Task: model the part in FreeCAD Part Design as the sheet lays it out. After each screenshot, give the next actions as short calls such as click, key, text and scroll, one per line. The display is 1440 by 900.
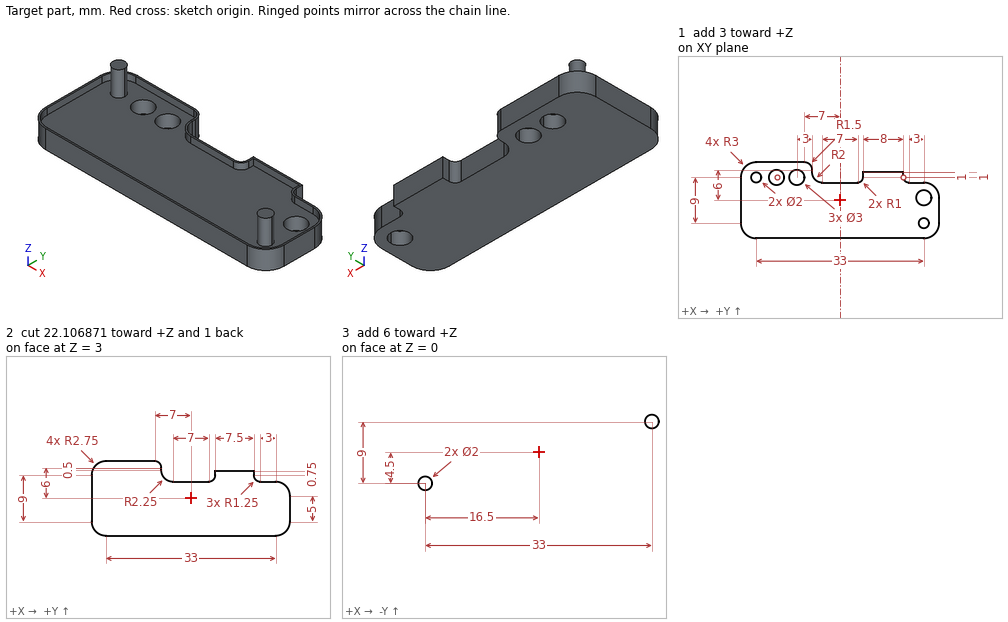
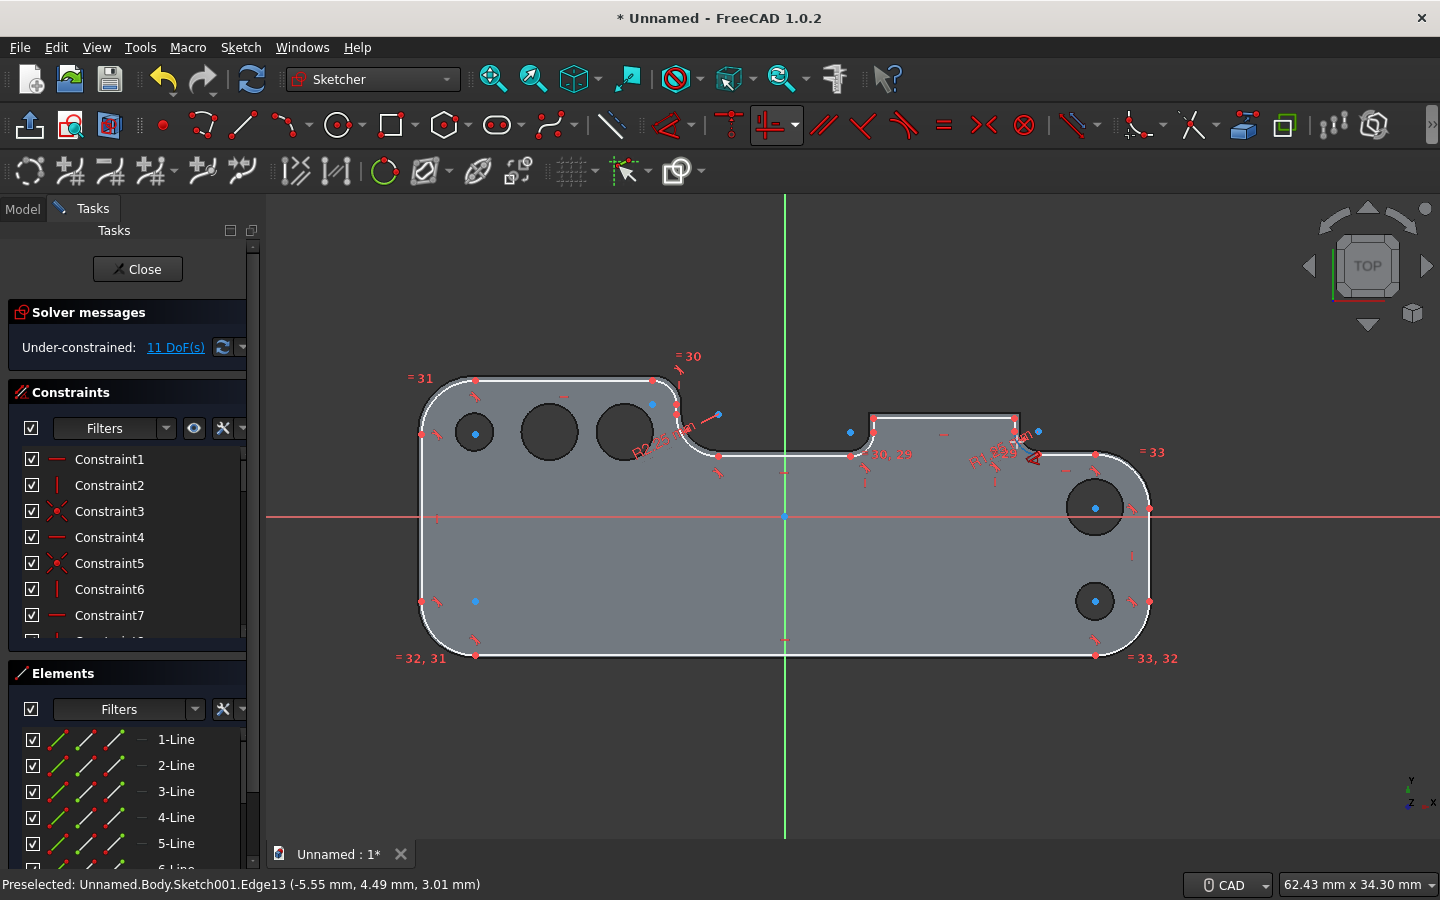
click(451, 387)
click(436, 359)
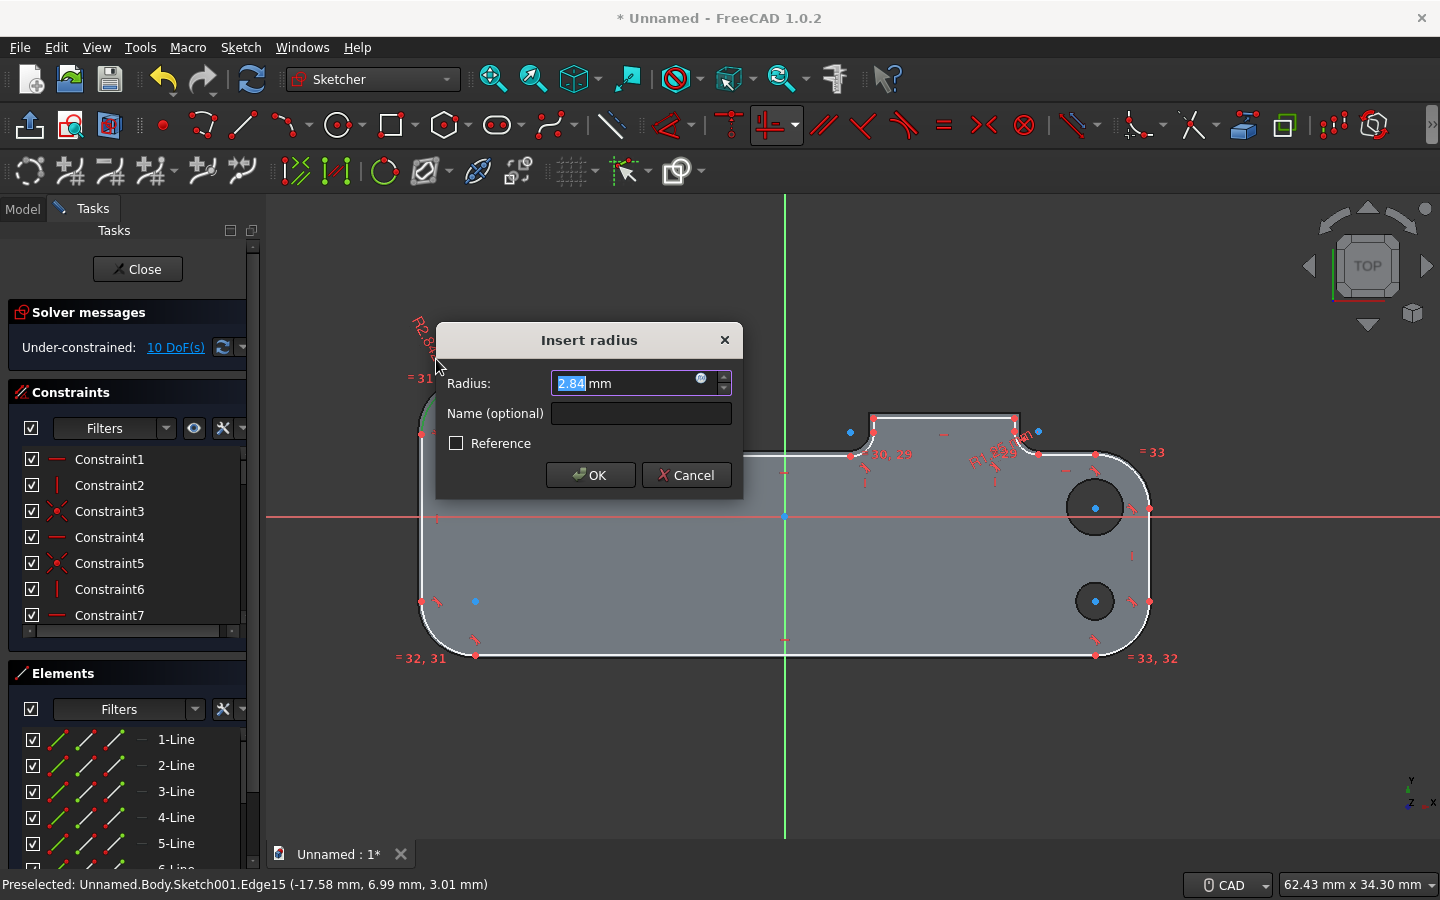
text(2.75)
key(Return)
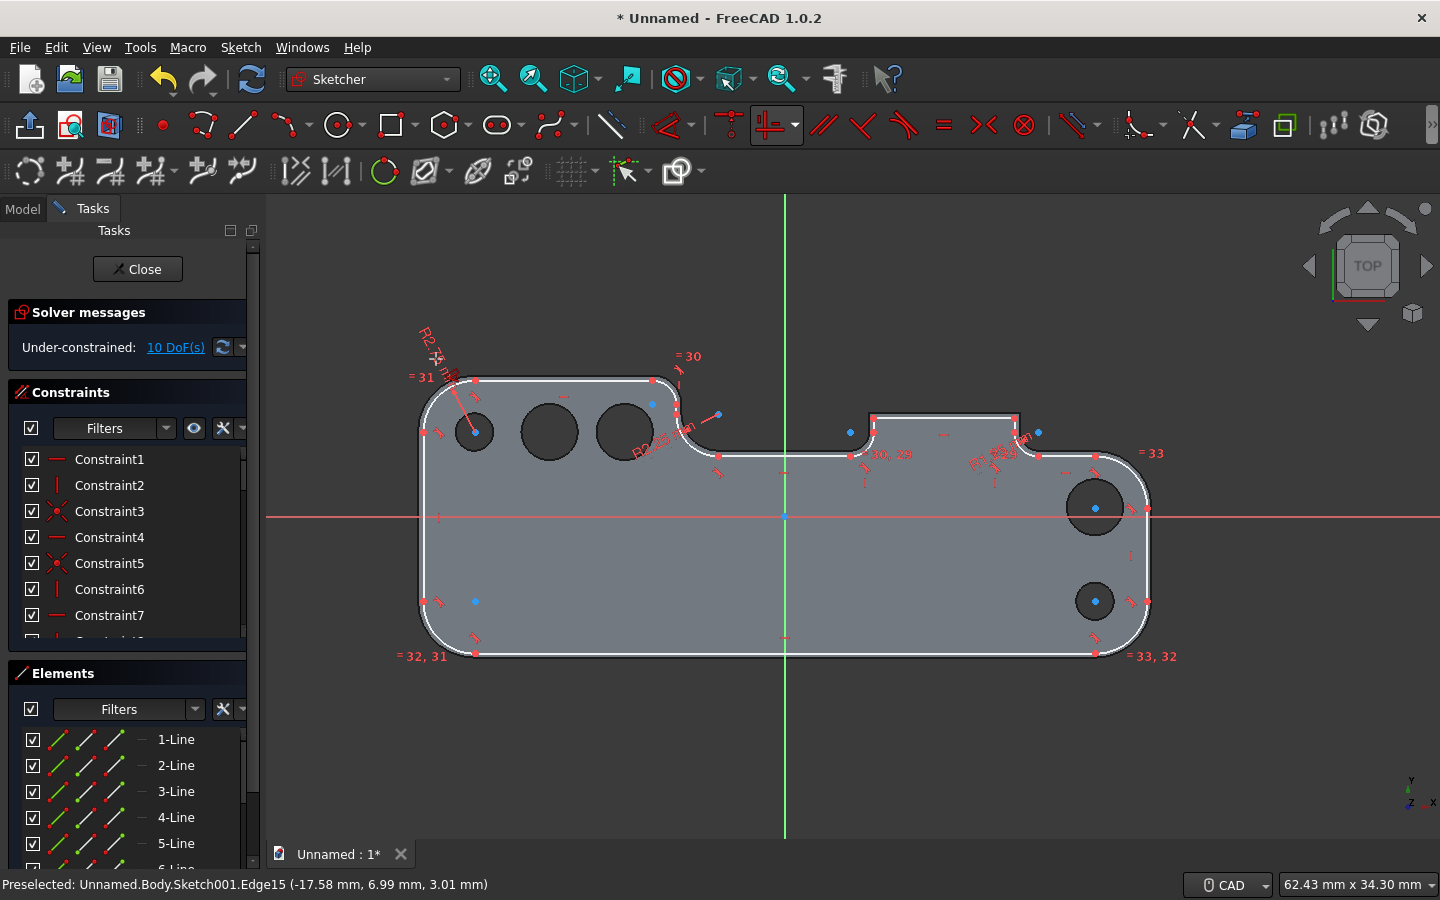
click(1078, 456)
click(1067, 422)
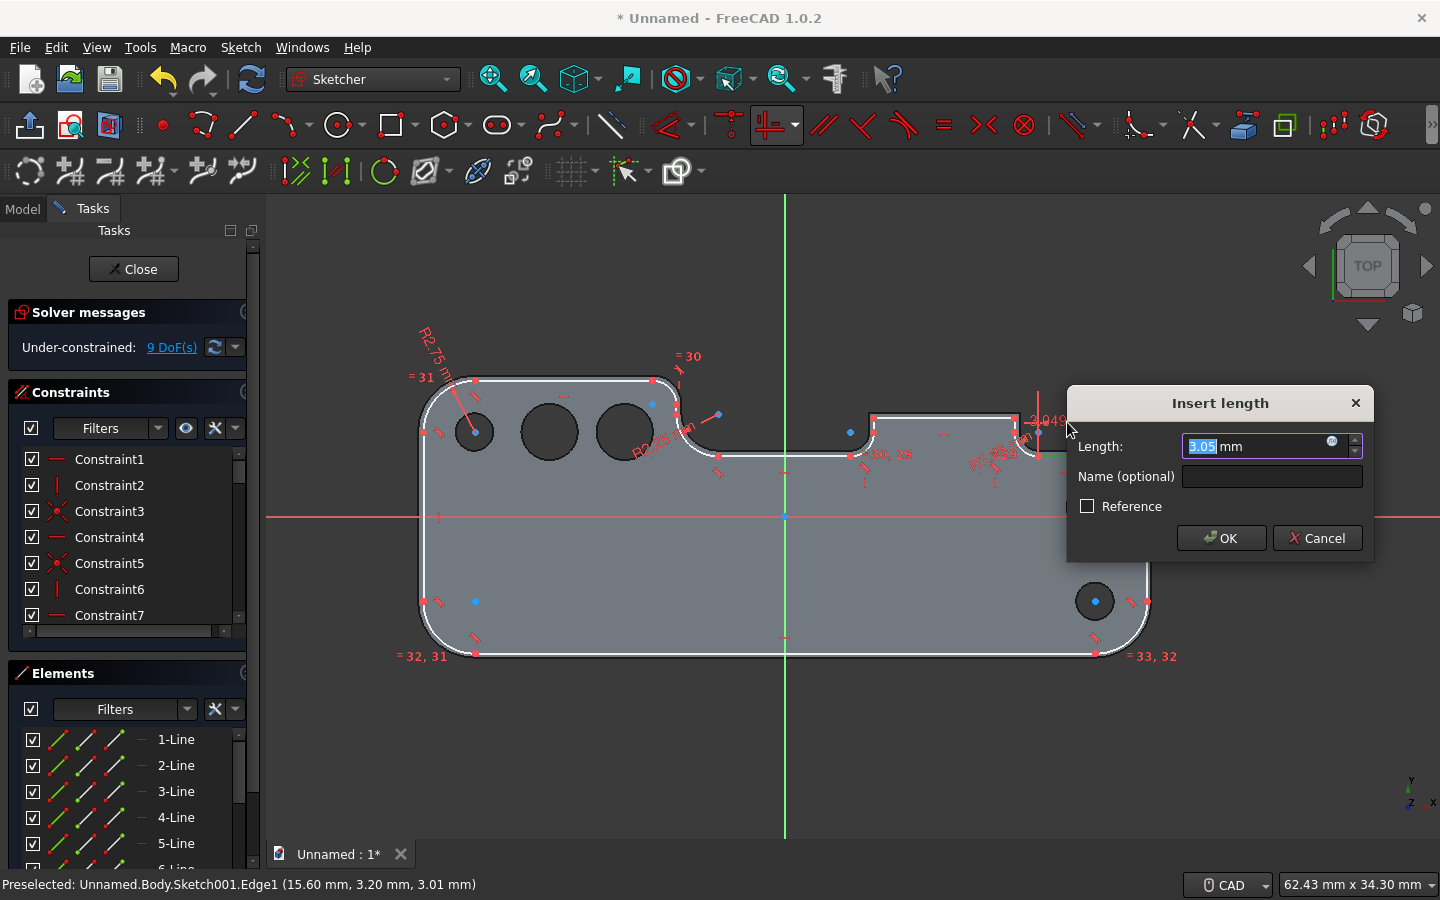
text(3)
key(Return)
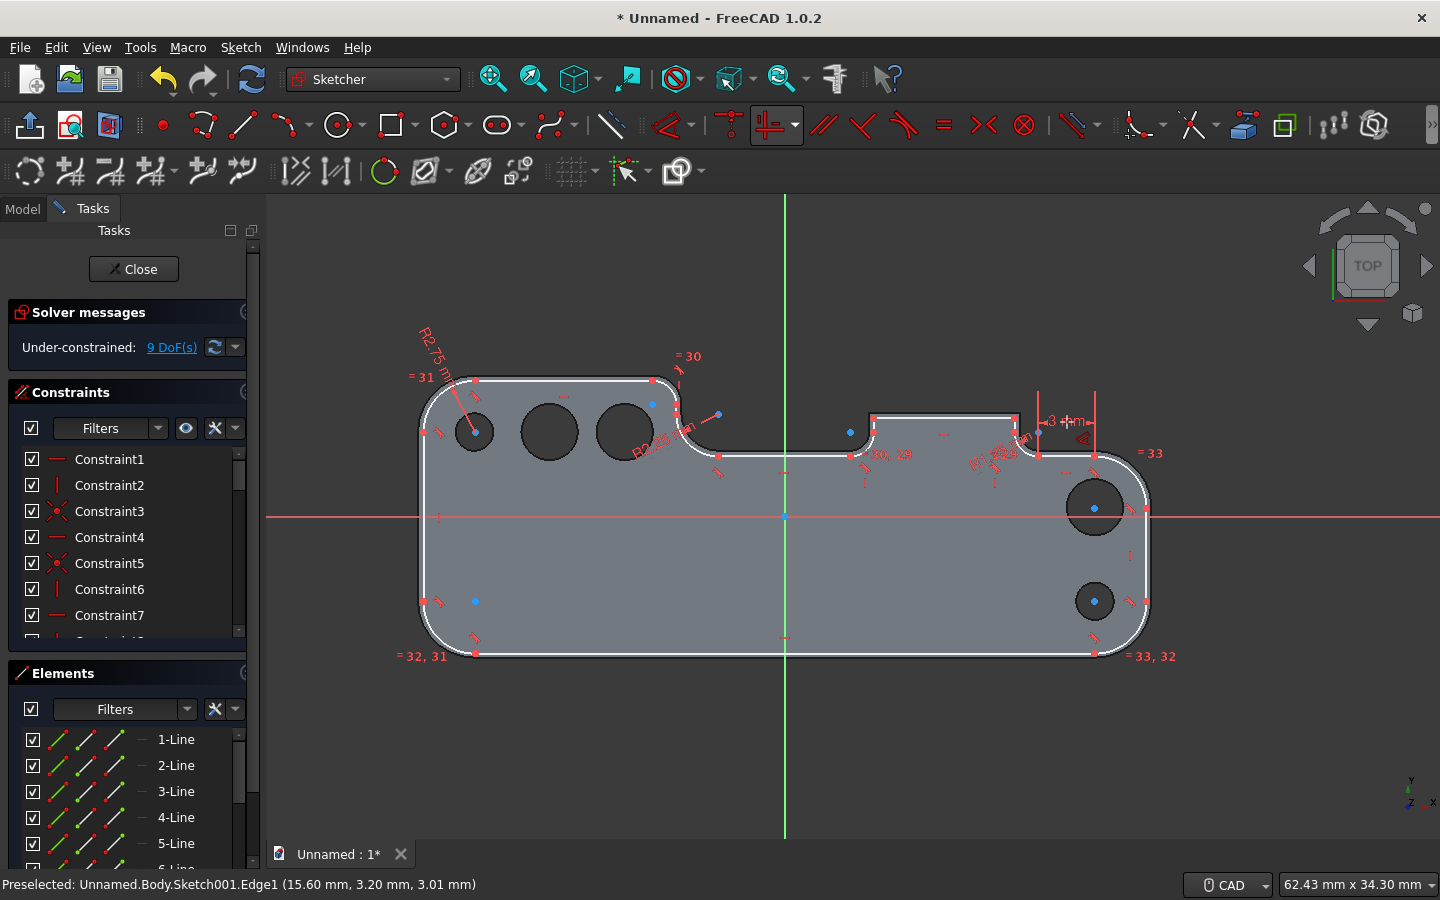
click(811, 456)
click(754, 422)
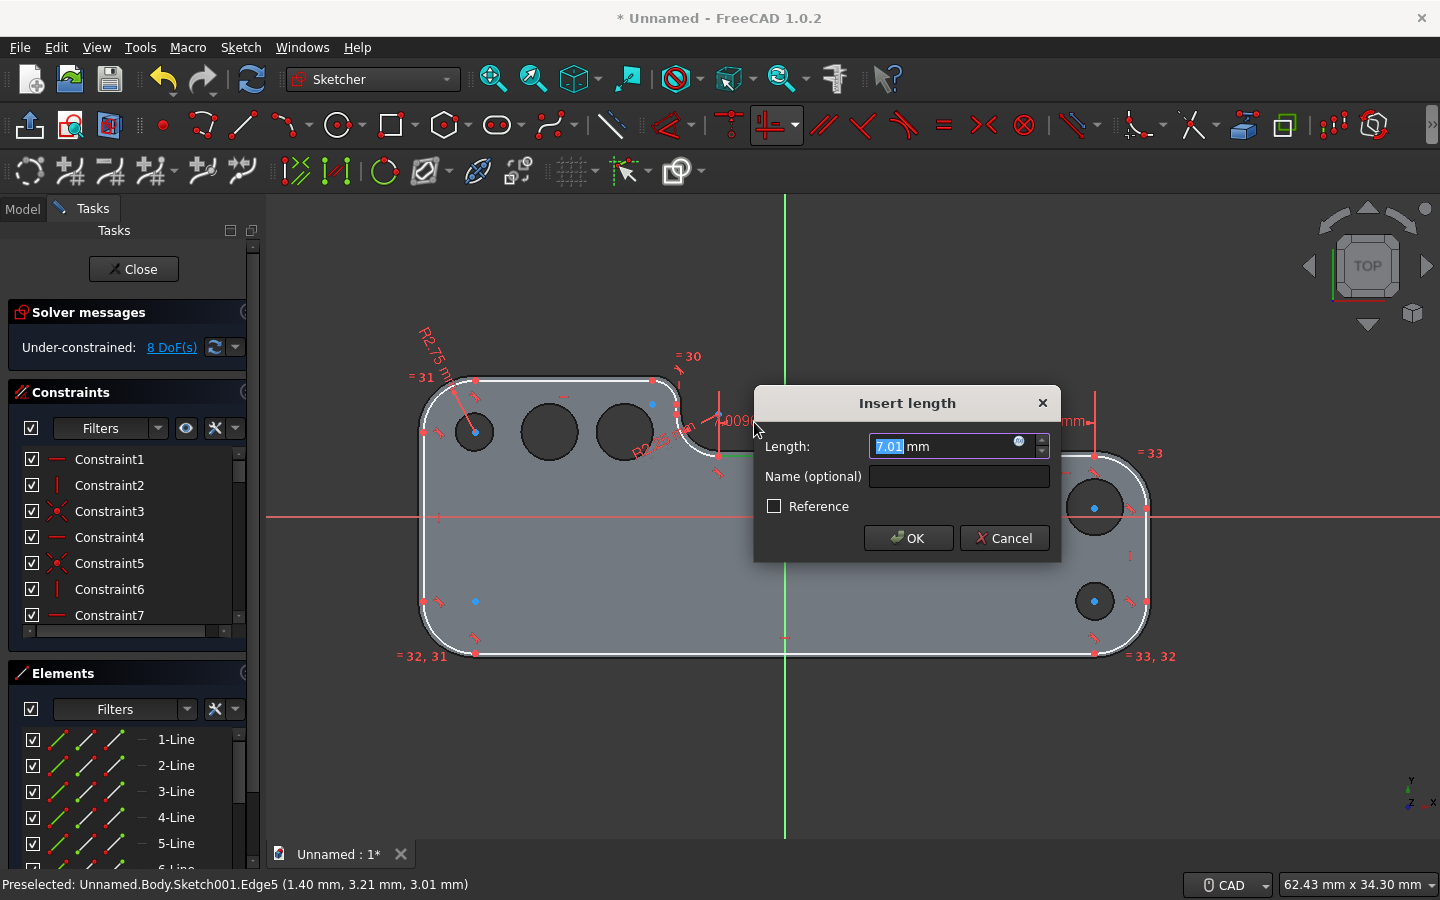
text(7)
key(Return)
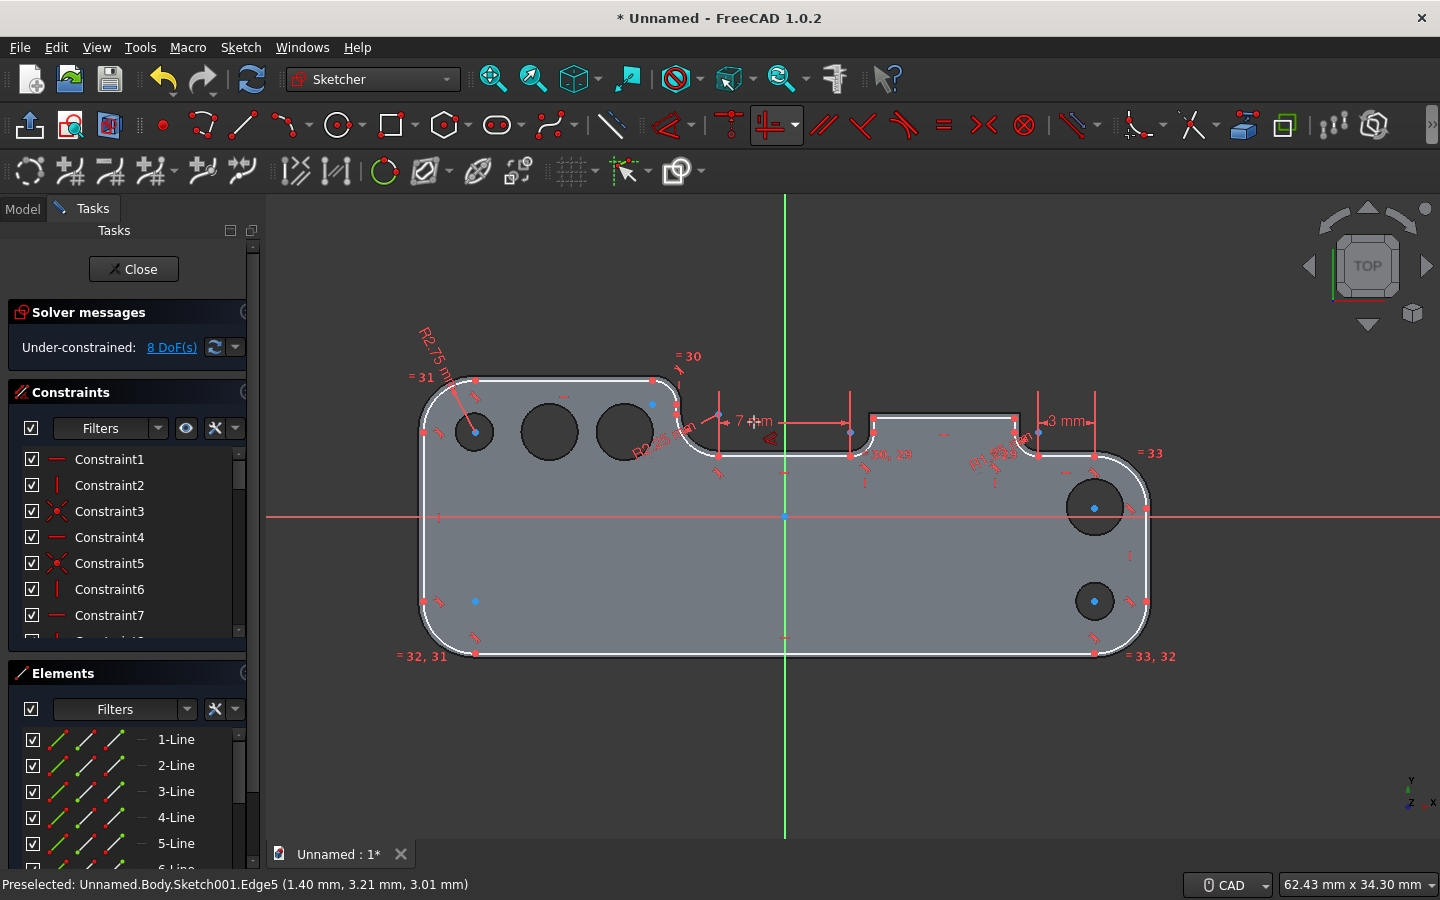
click(424, 483)
click(390, 478)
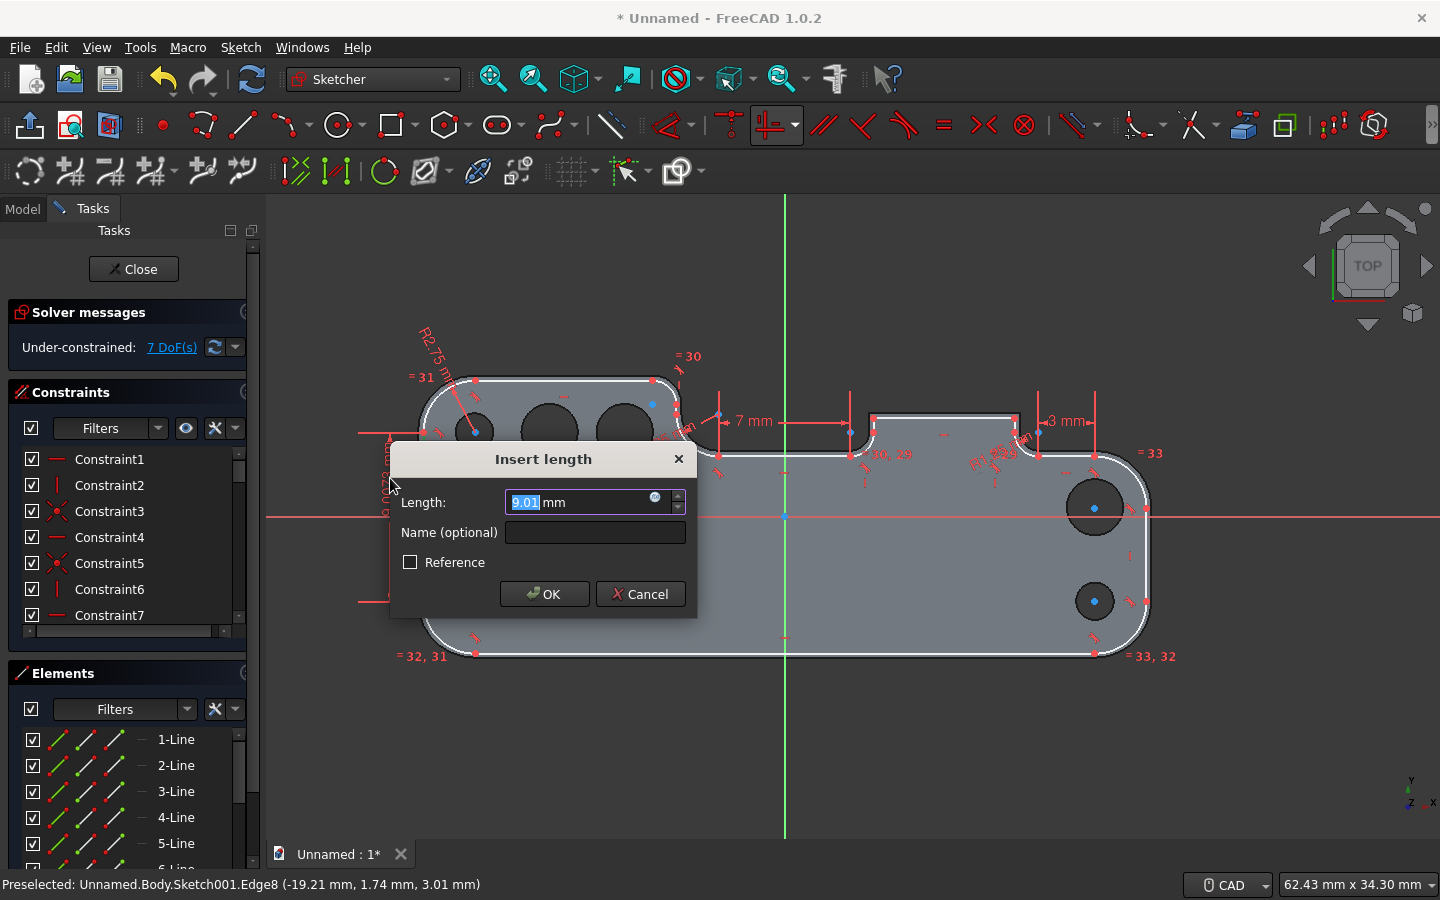
text(9)
key(Return)